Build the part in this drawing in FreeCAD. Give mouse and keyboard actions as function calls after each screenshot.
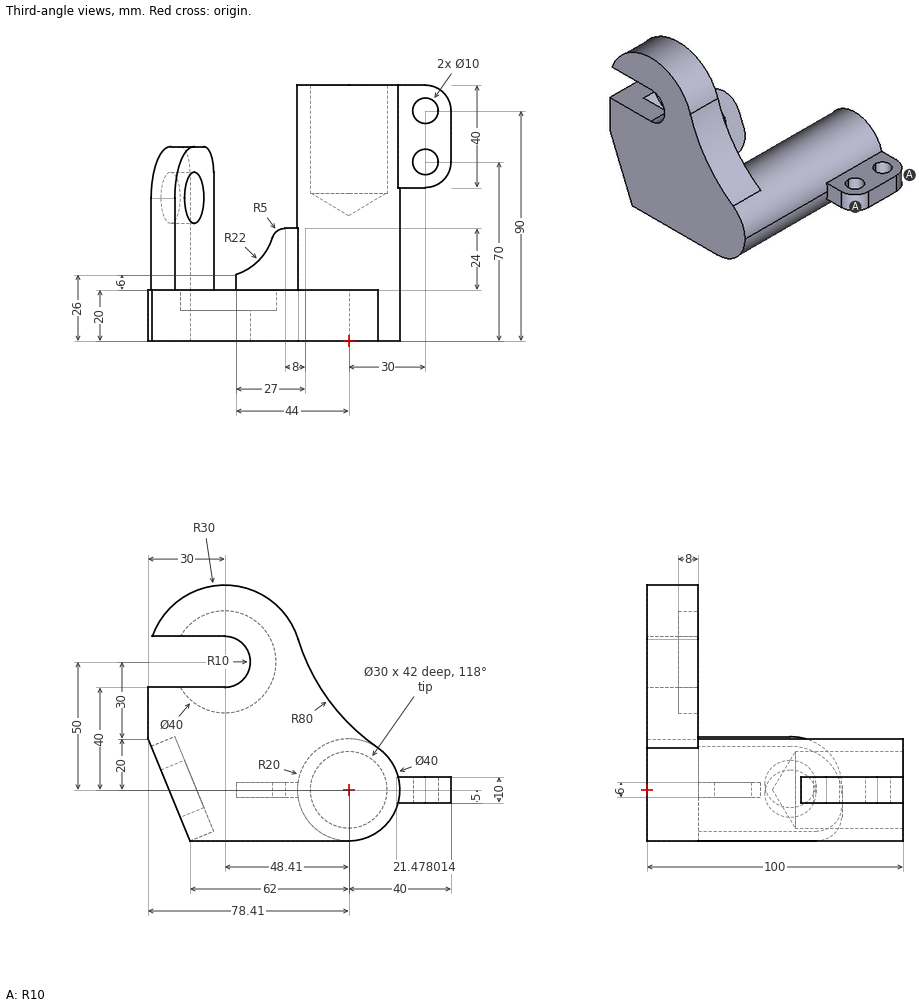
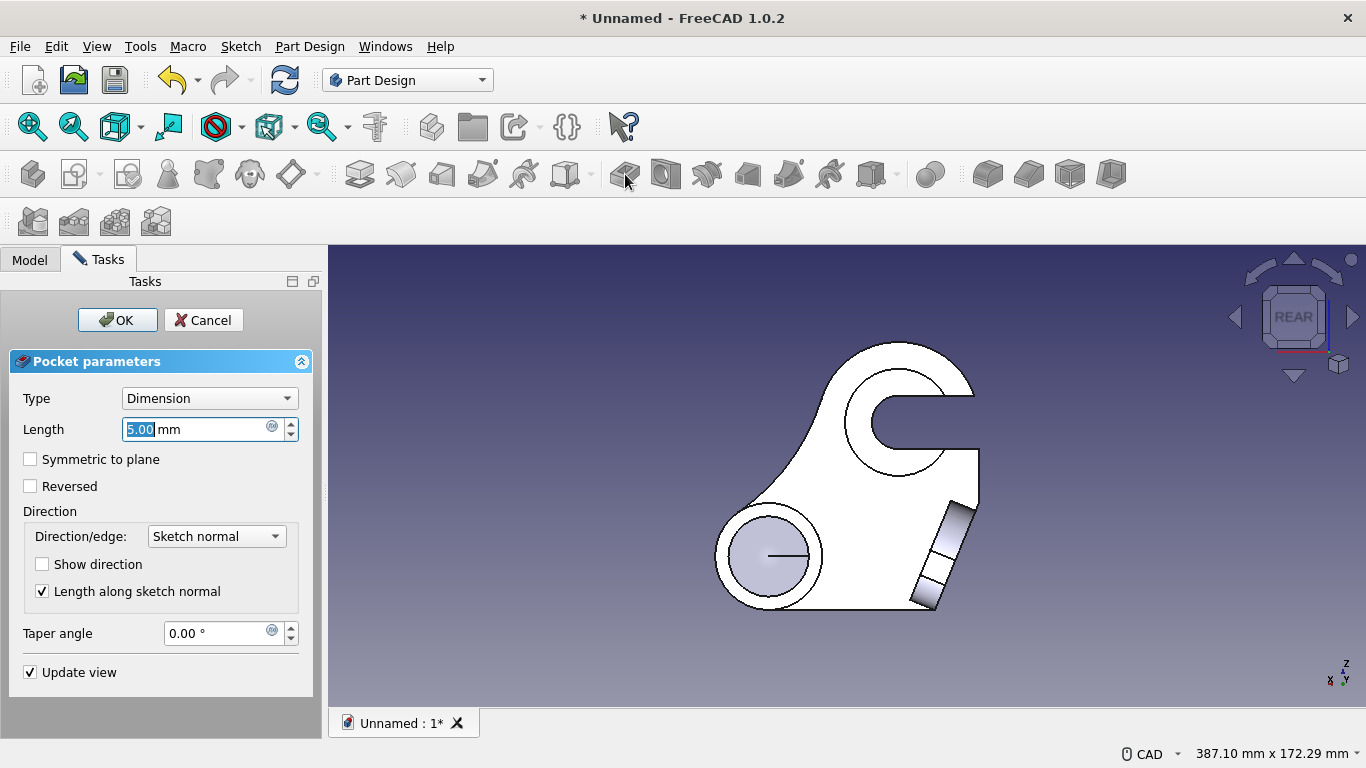
text(8)
key(Tab)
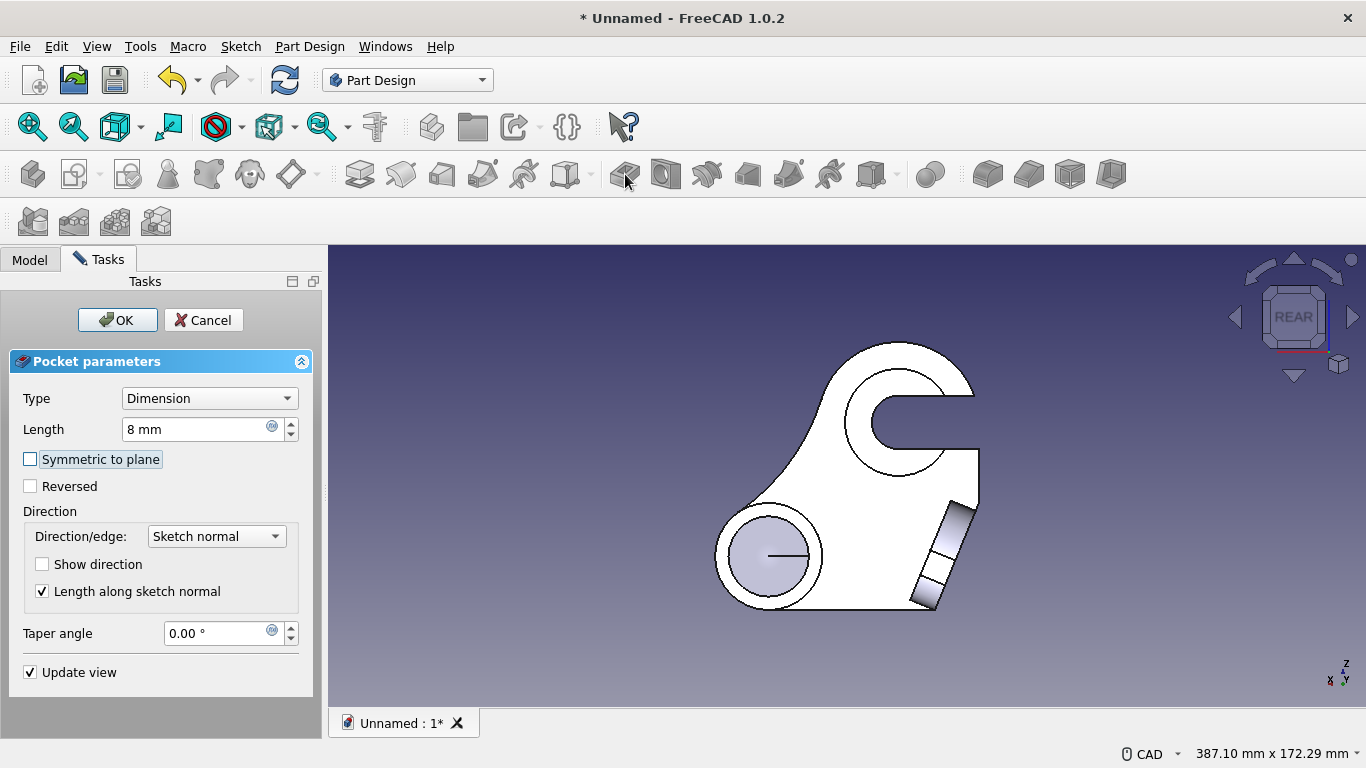
click(118, 320)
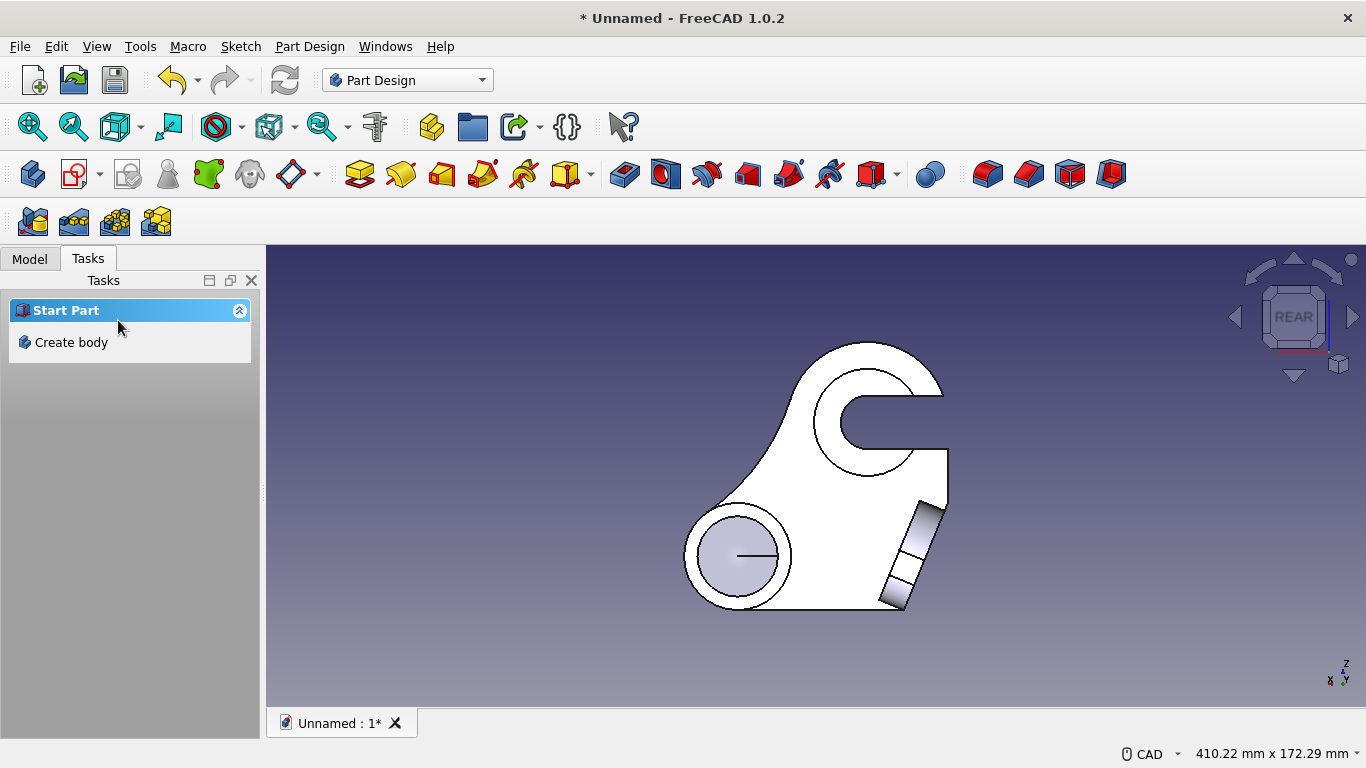
scroll(738, 601, up, 4)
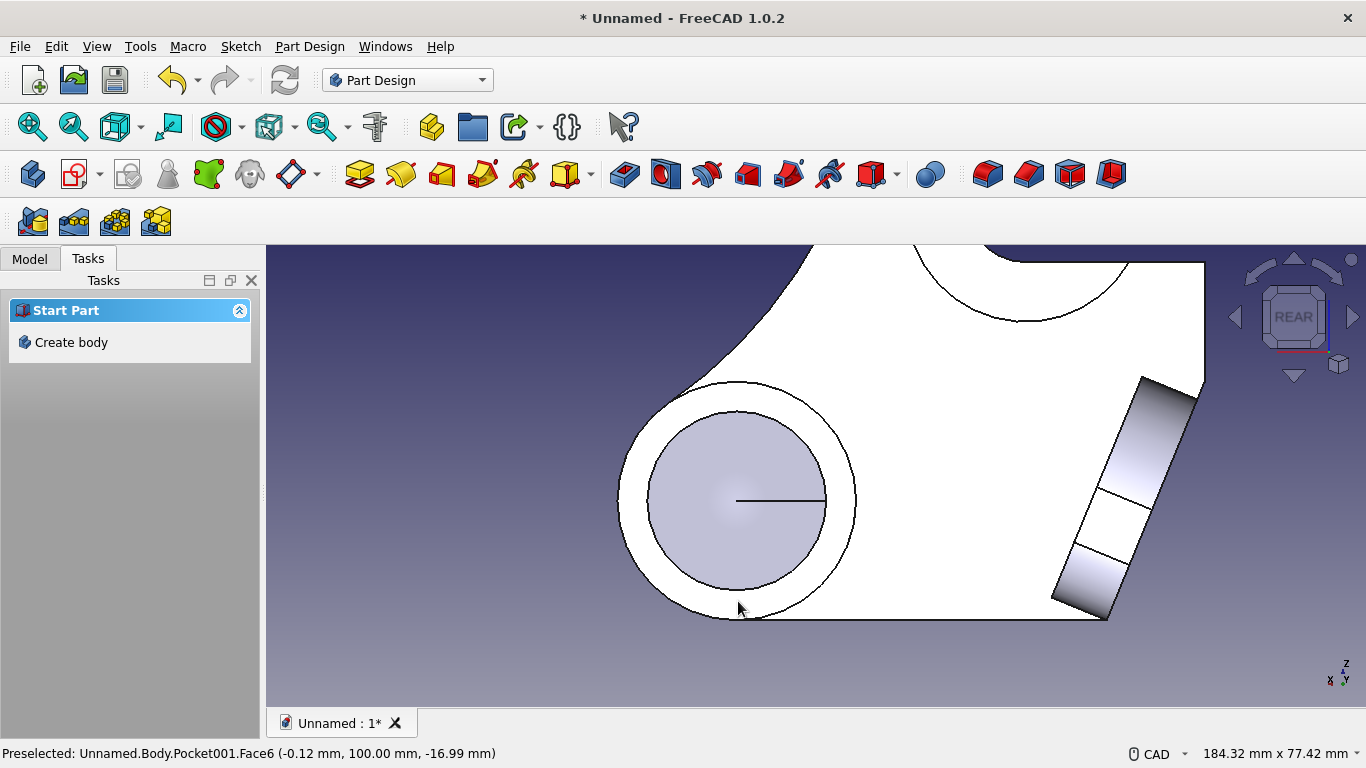
click(737, 602)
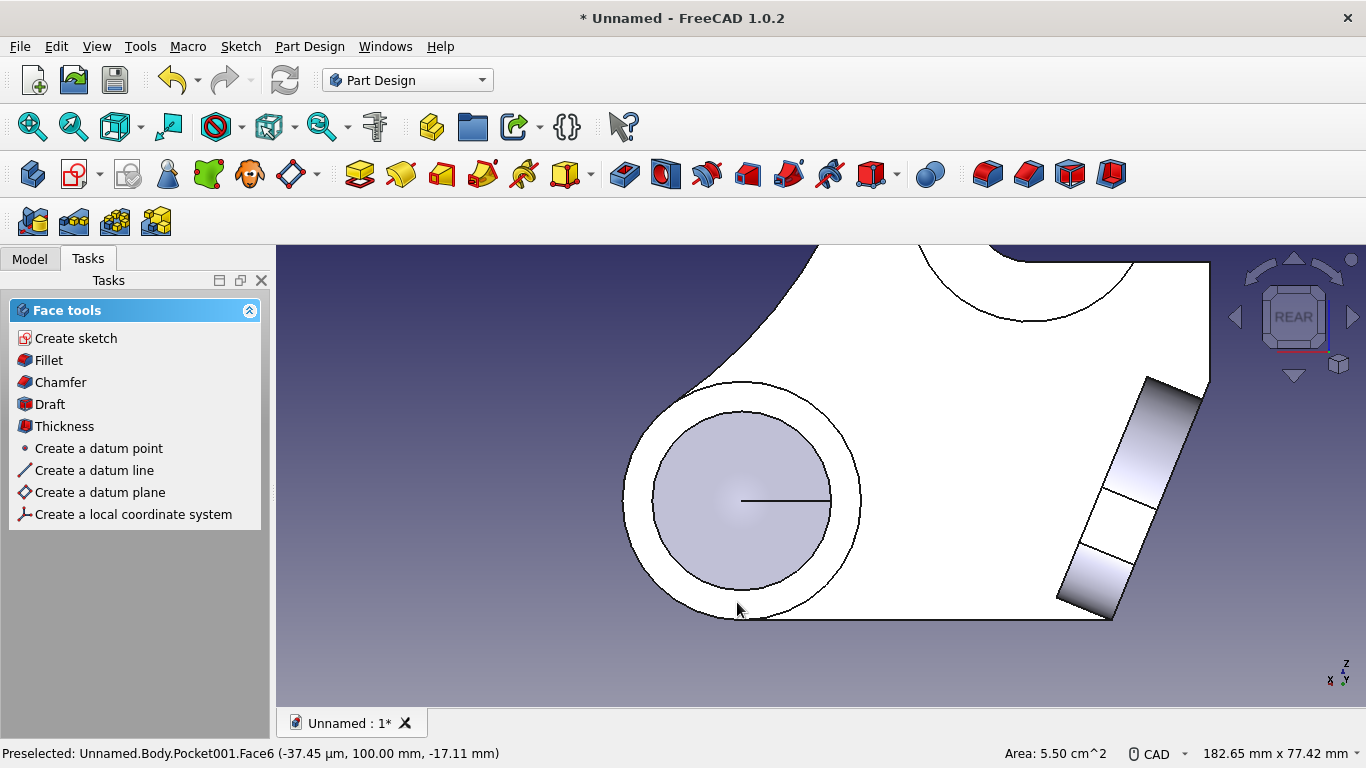
click(74, 174)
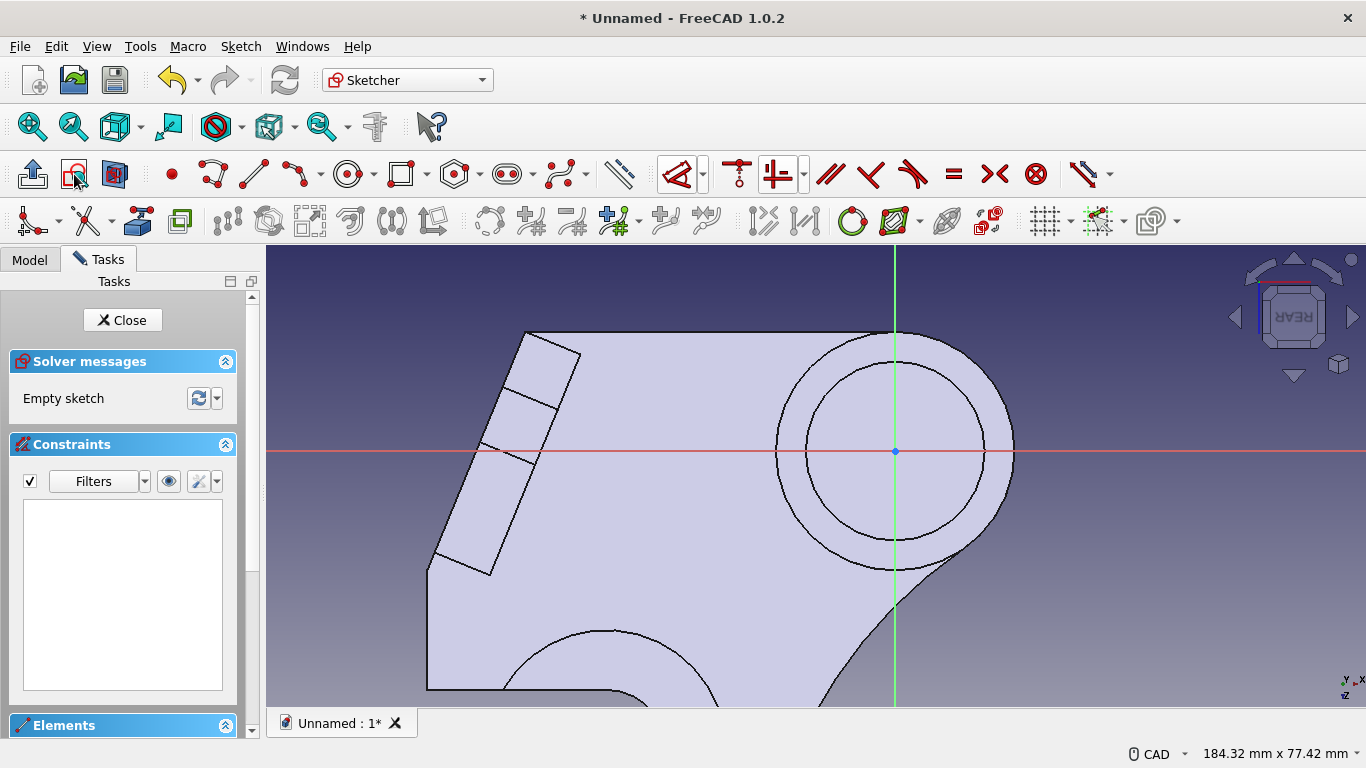
scroll(1170, 437, up, 5)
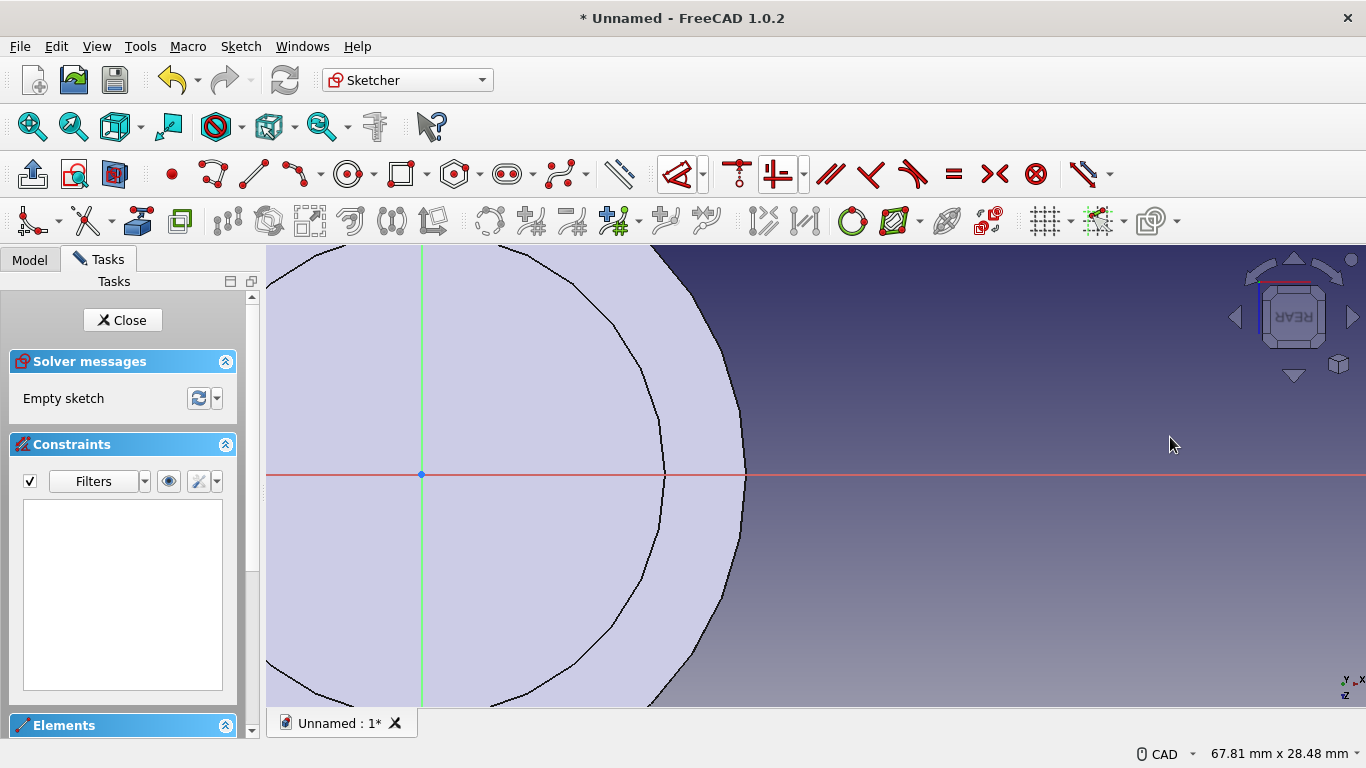
click(400, 174)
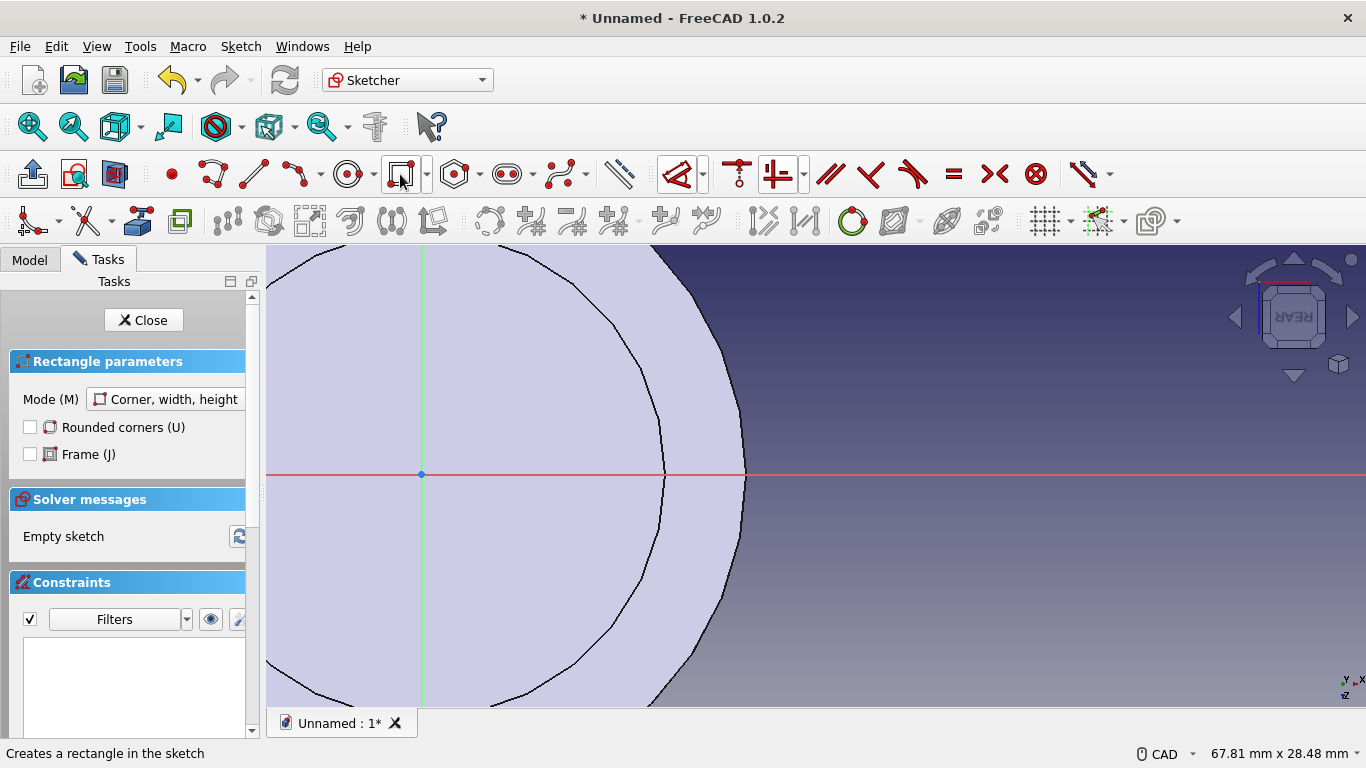
click(722, 394)
click(1071, 556)
key(Escape)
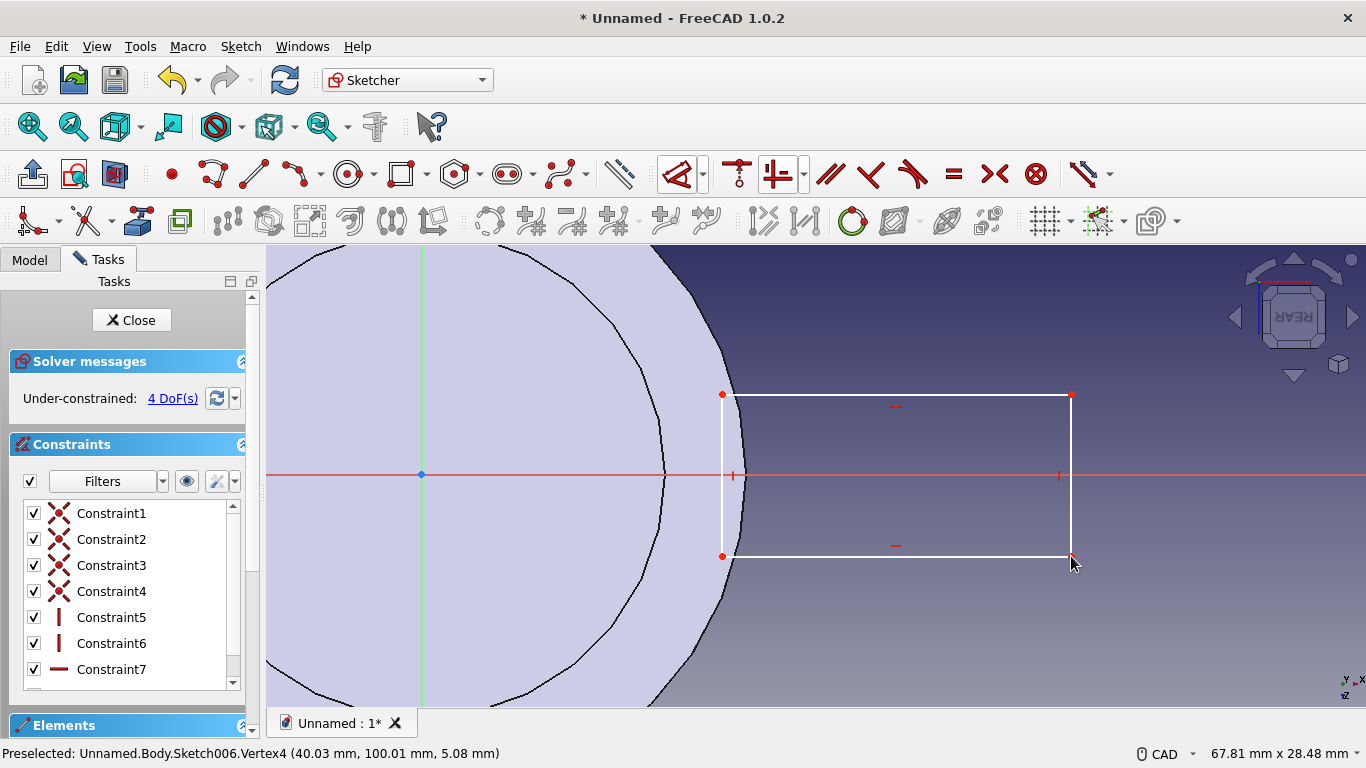
key(d)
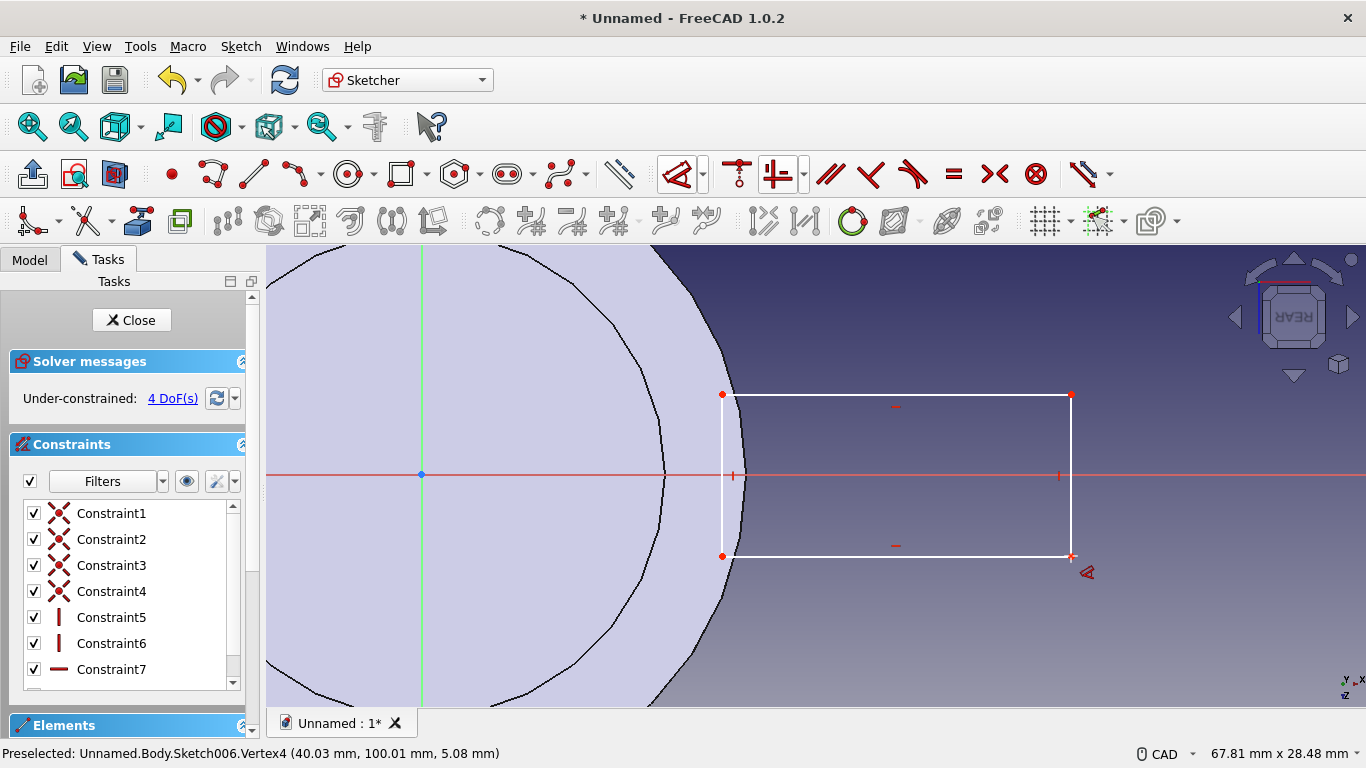
click(722, 444)
click(688, 439)